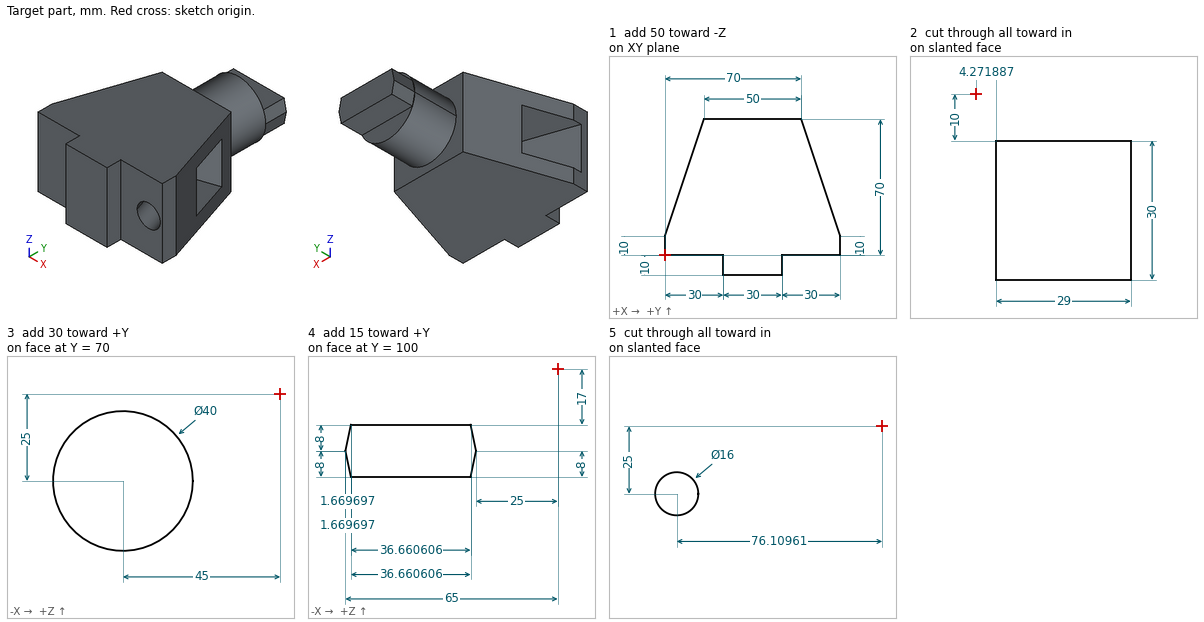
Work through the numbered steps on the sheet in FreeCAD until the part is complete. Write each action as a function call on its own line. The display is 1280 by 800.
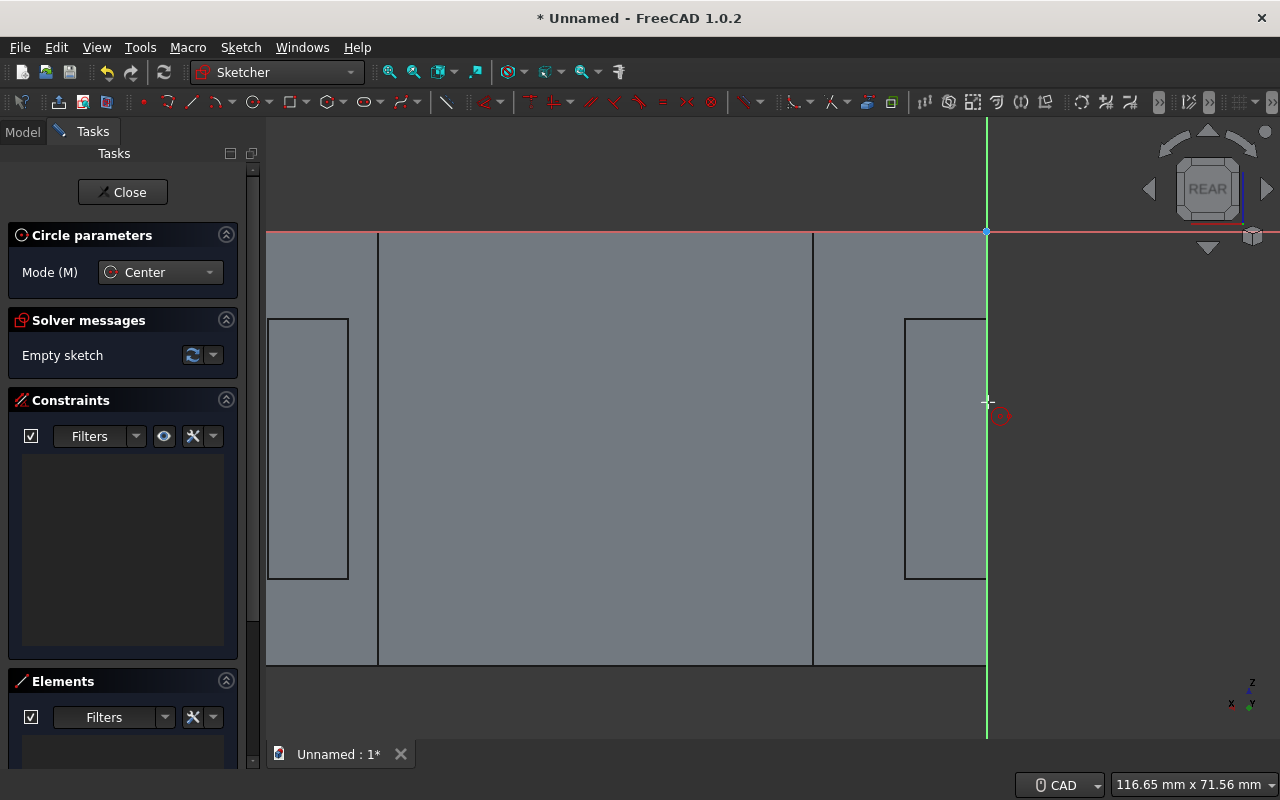
click(596, 449)
move(719, 326)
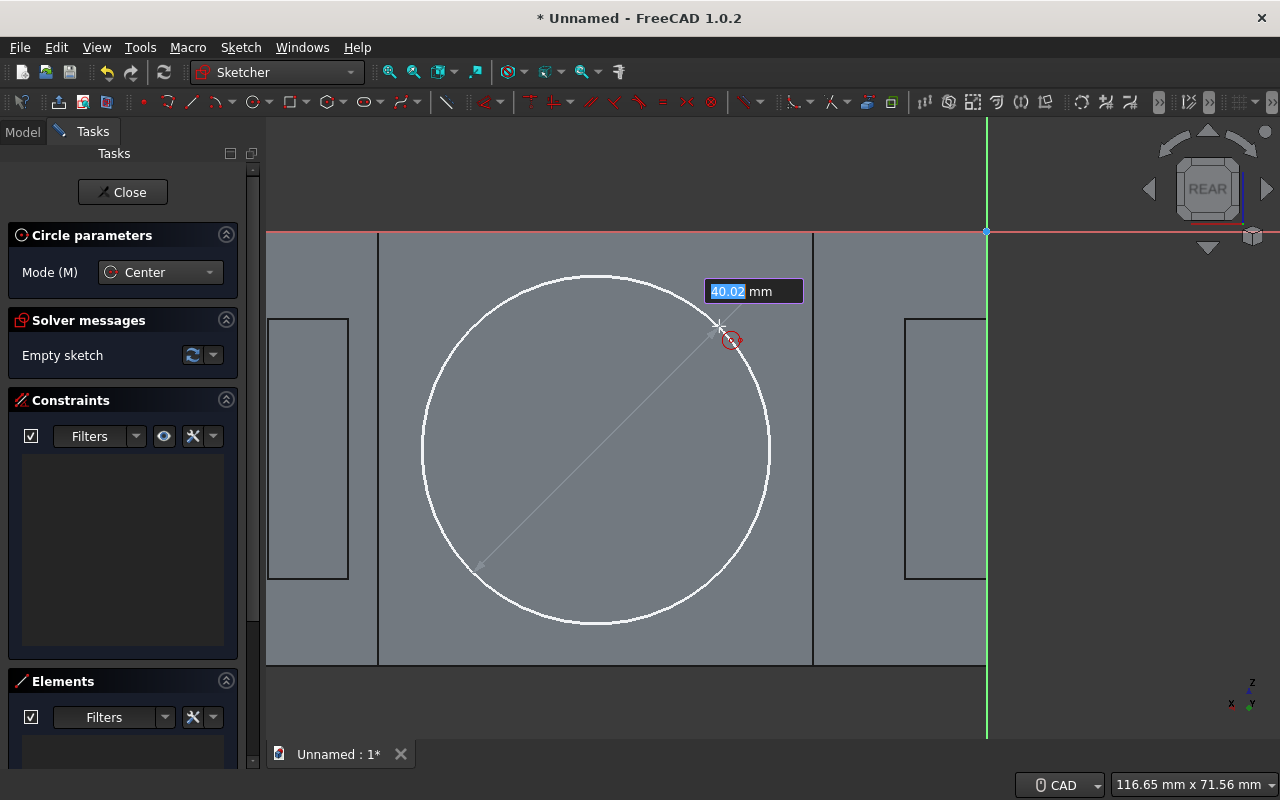
text(40)
key(Return)
key(Escape)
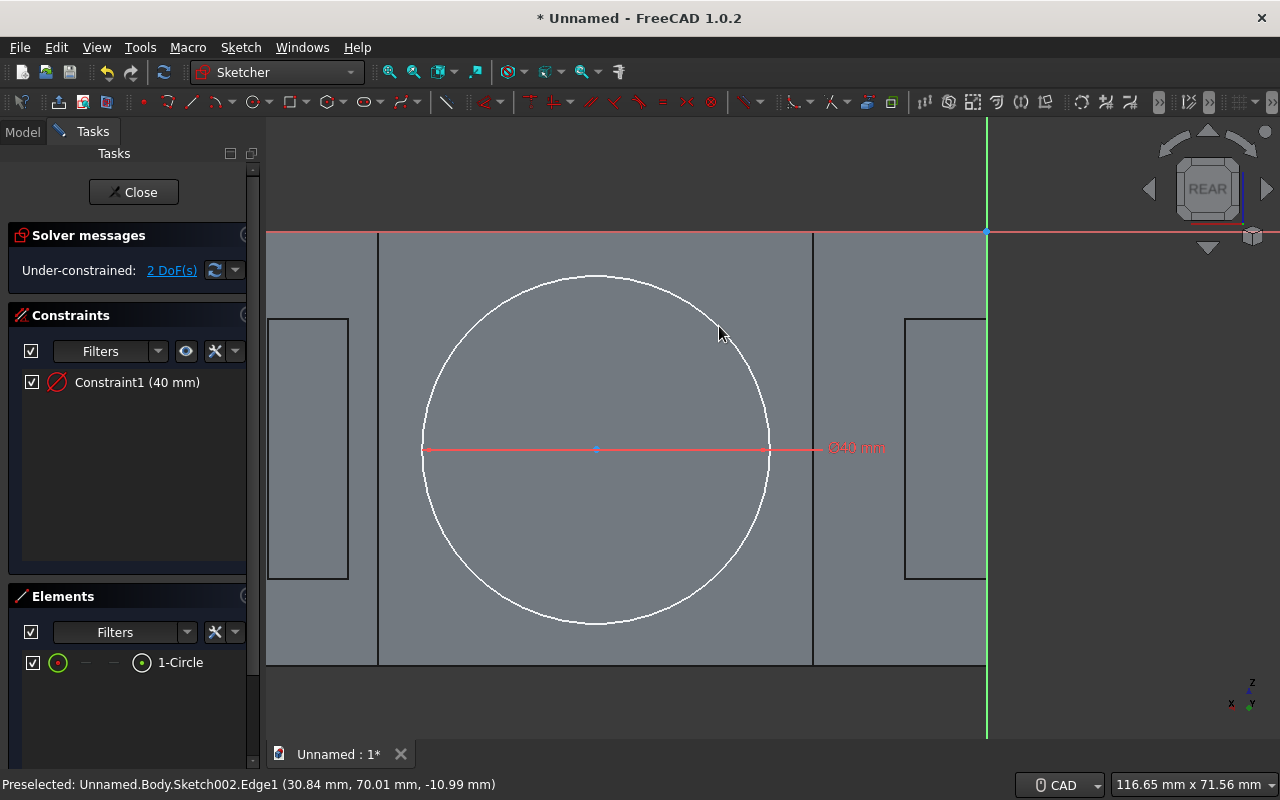
click(484, 102)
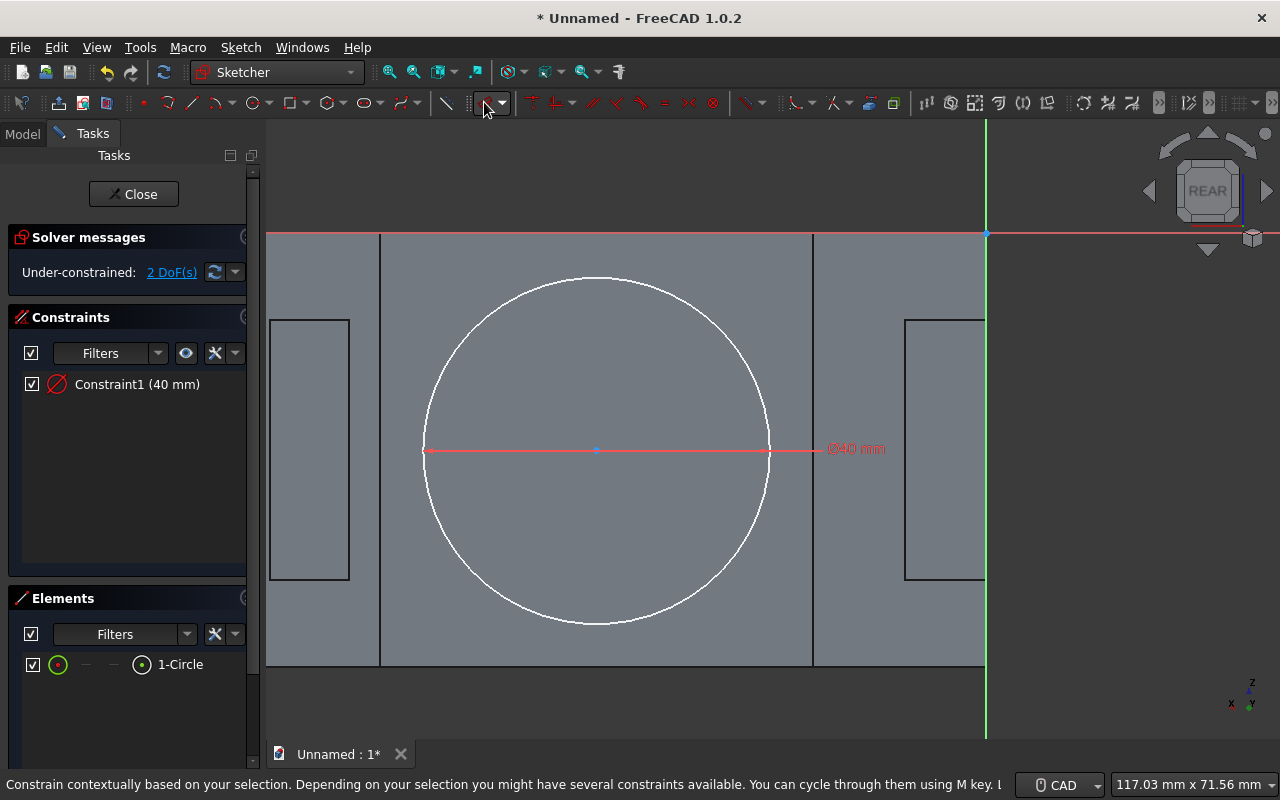
click(597, 451)
click(791, 199)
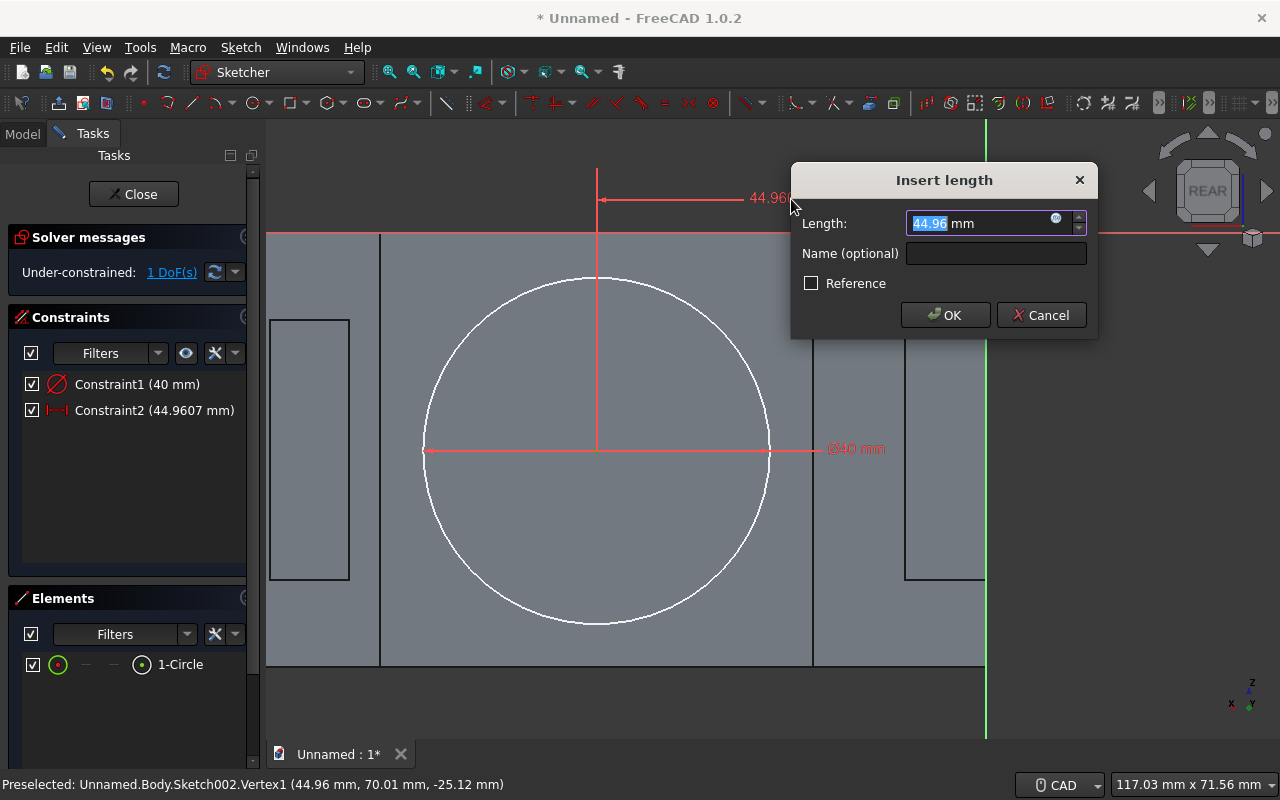
text(45)
key(Return)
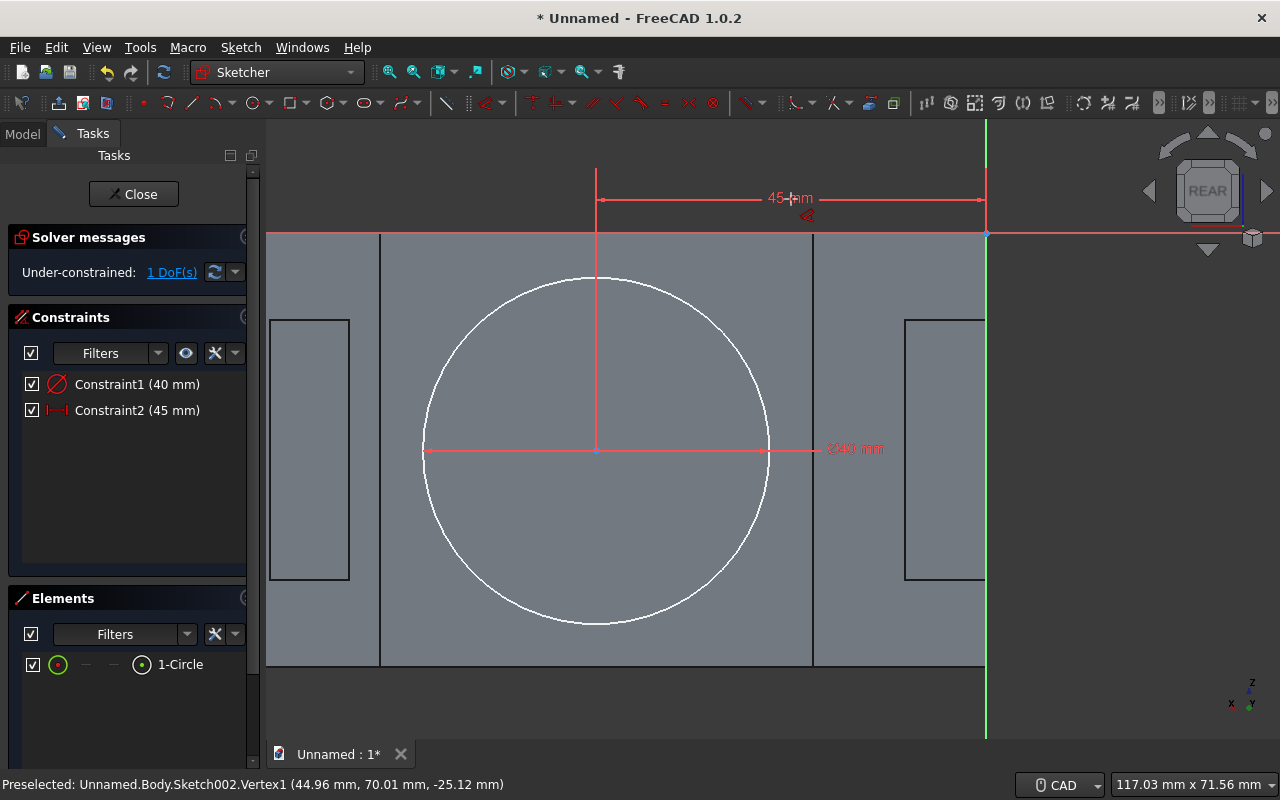
click(596, 451)
click(1020, 342)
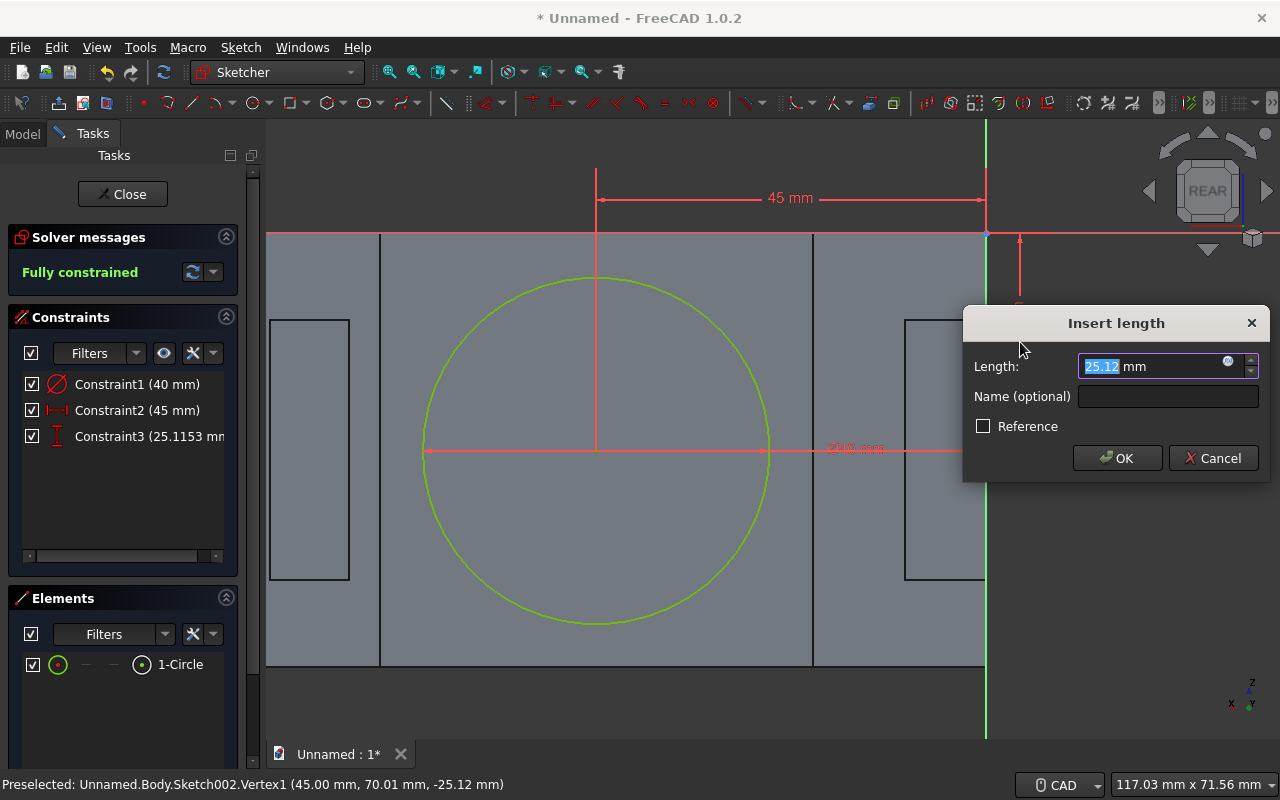
text(25)
key(Return)
key(Escape)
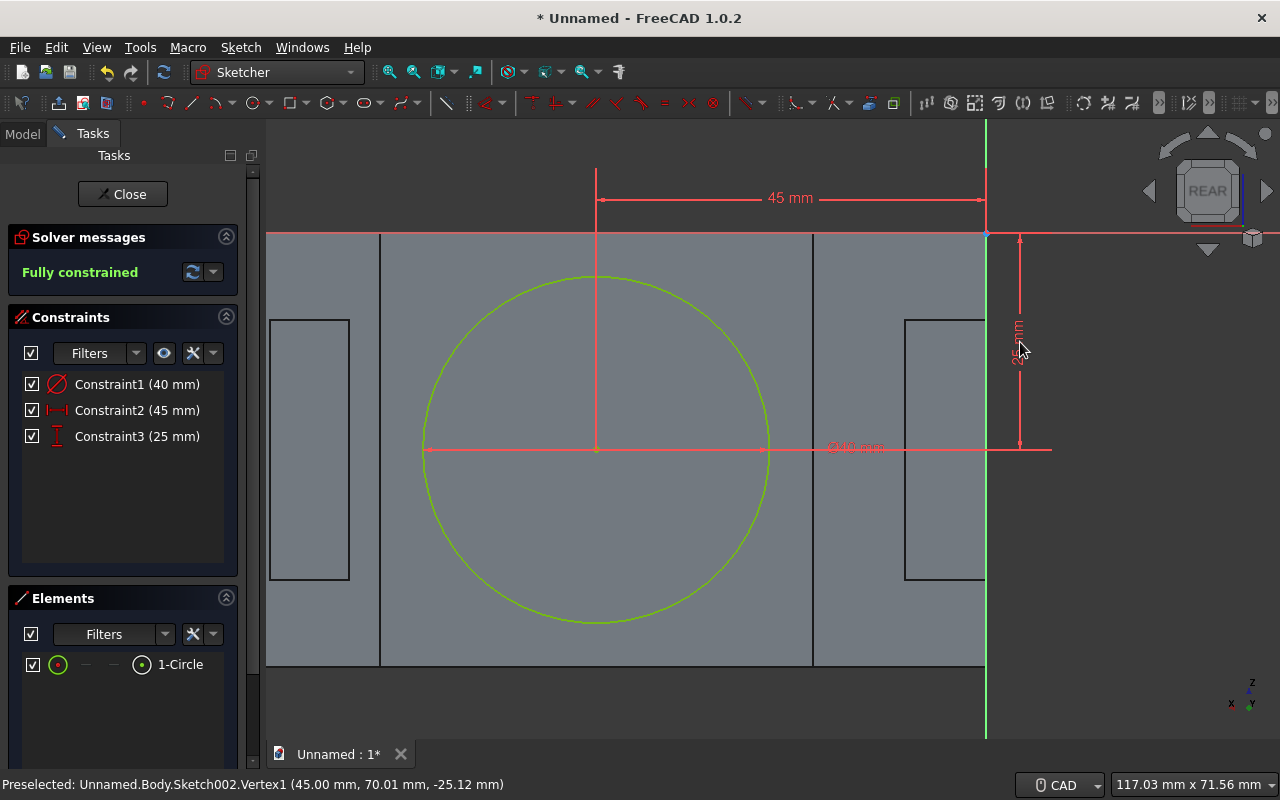
click(123, 194)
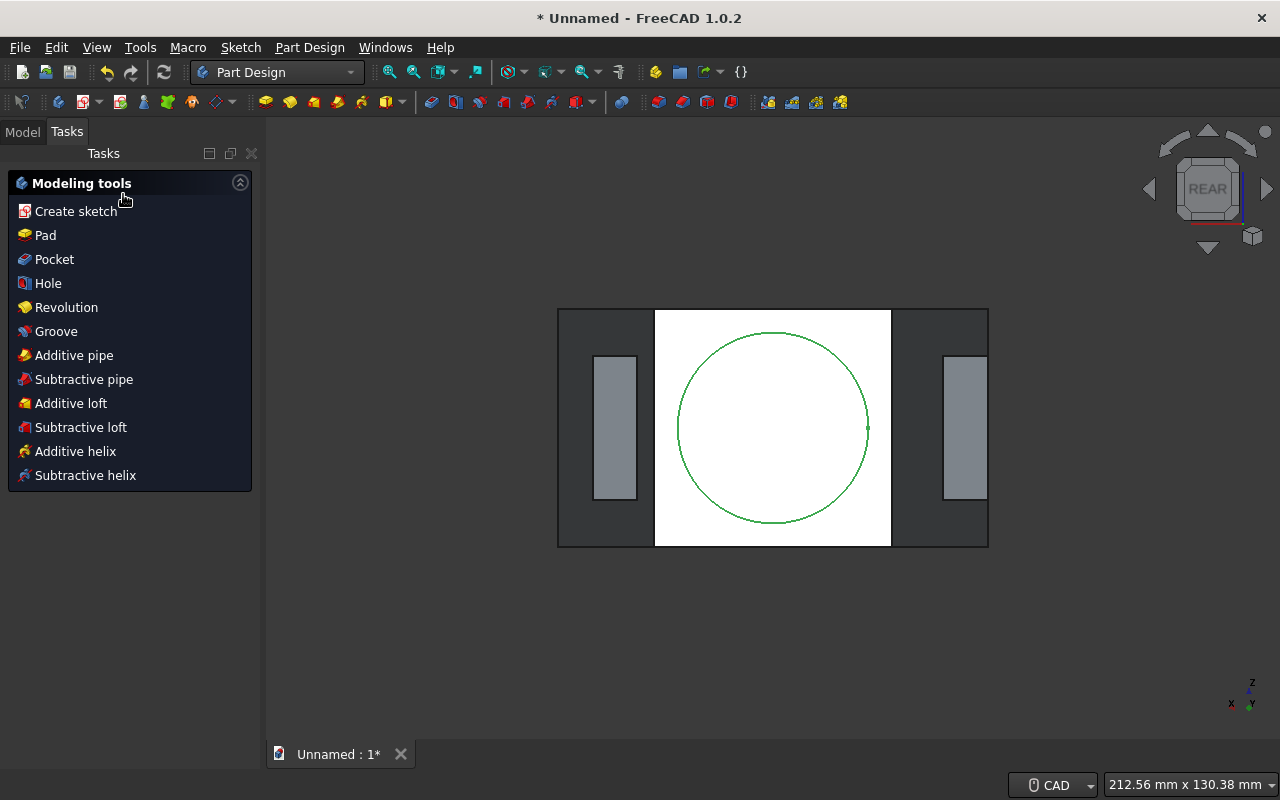
click(266, 102)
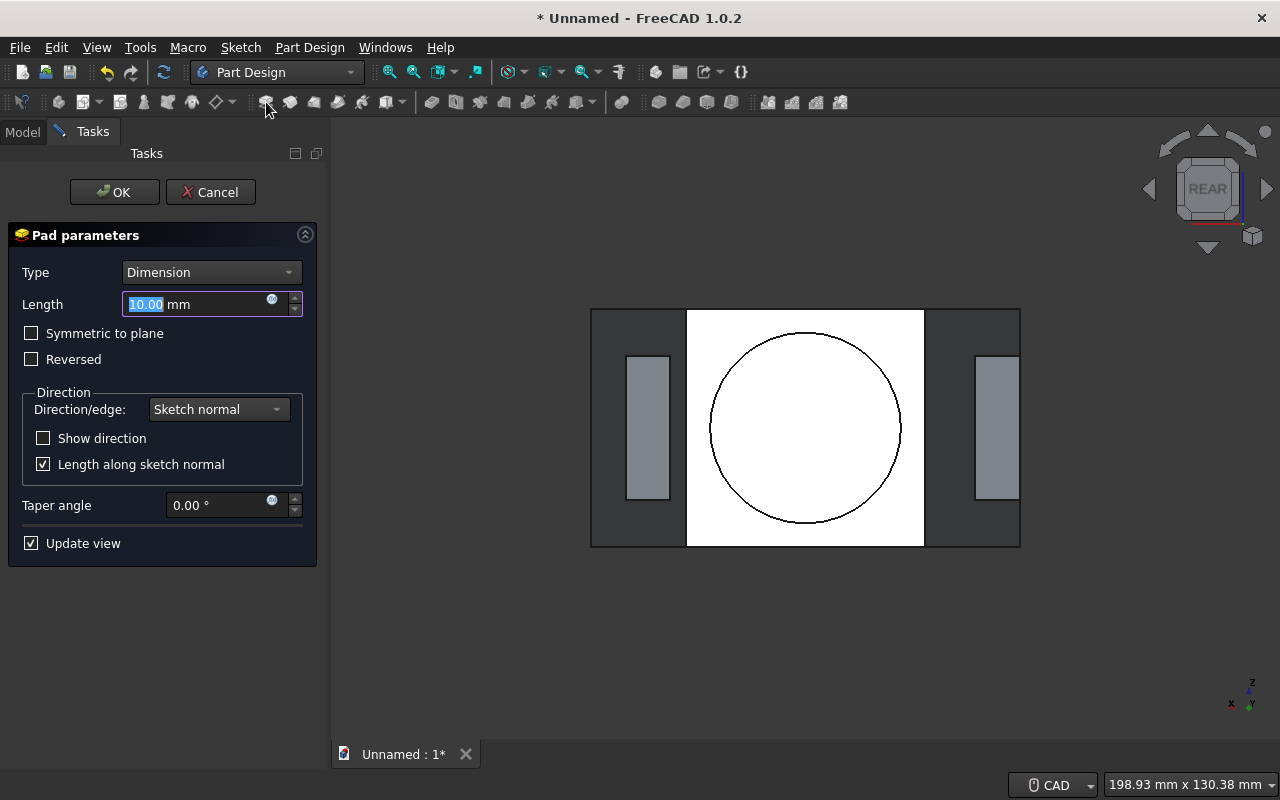
text(30)
key(Tab)